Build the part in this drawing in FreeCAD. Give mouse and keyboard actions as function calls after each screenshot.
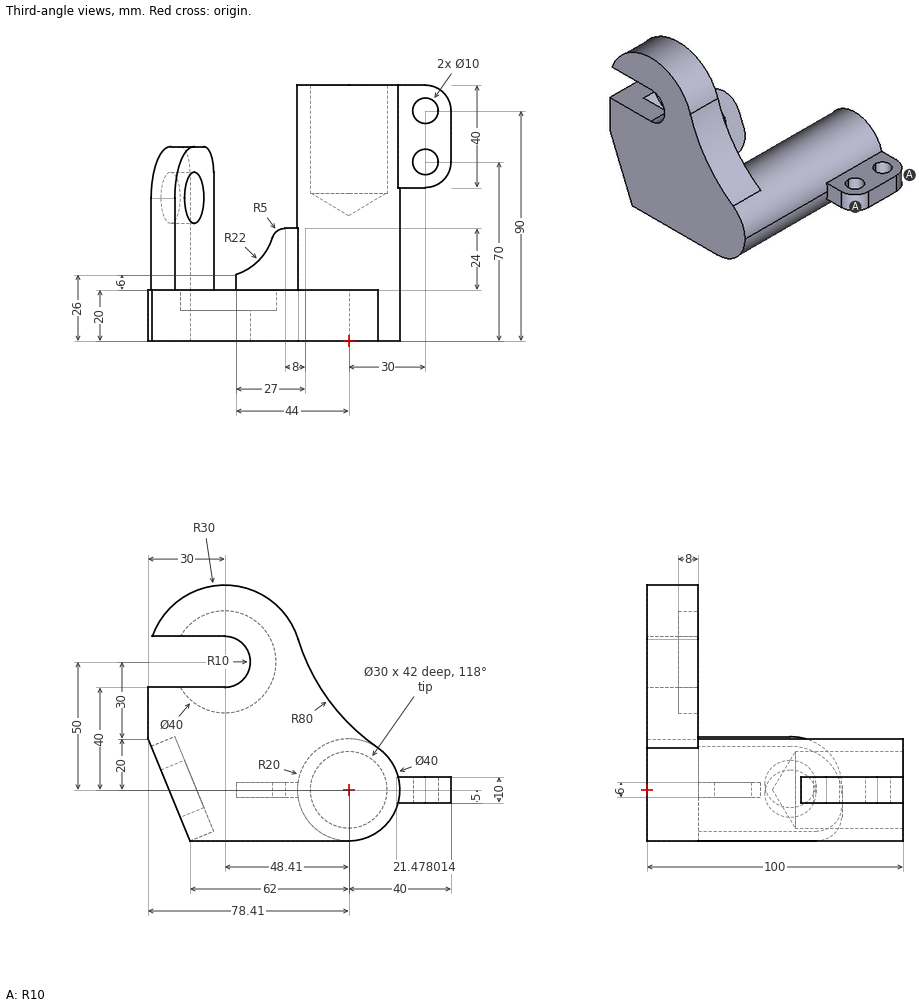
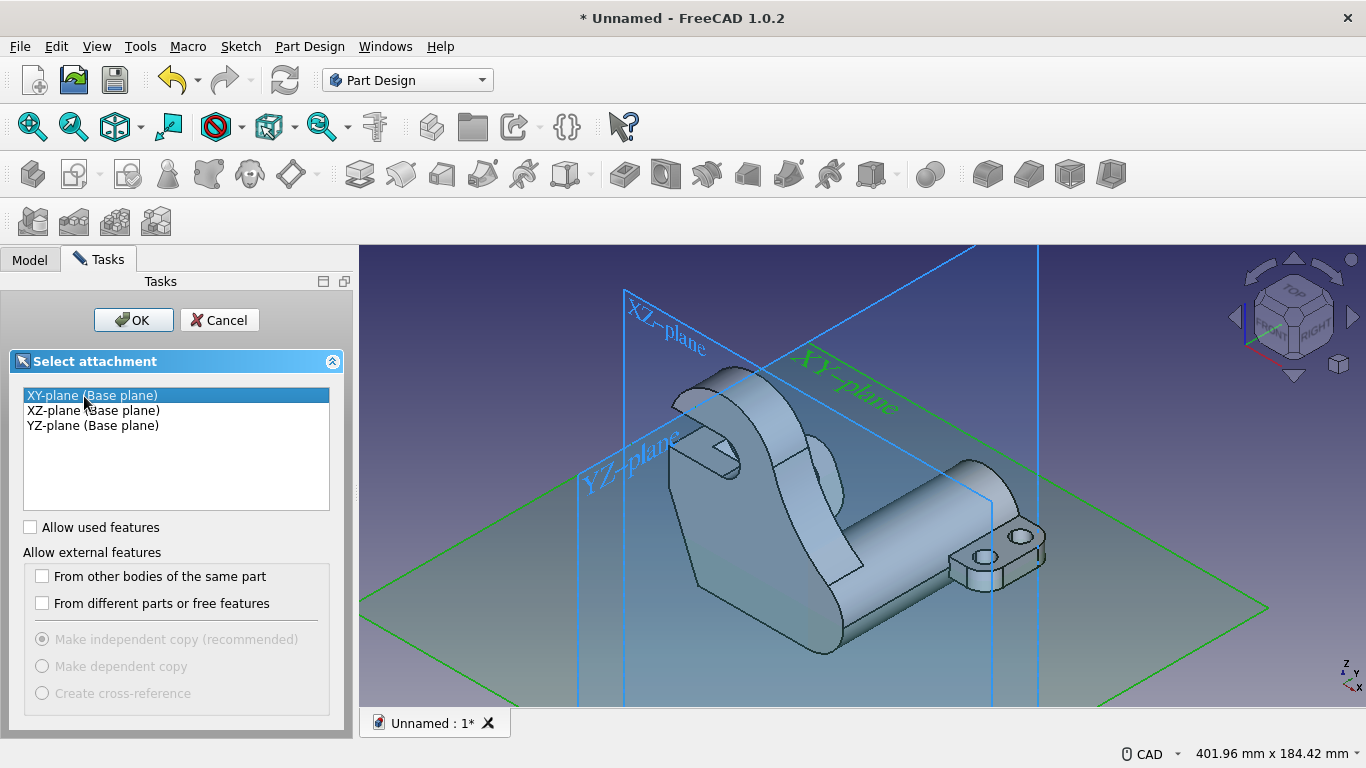
click(134, 320)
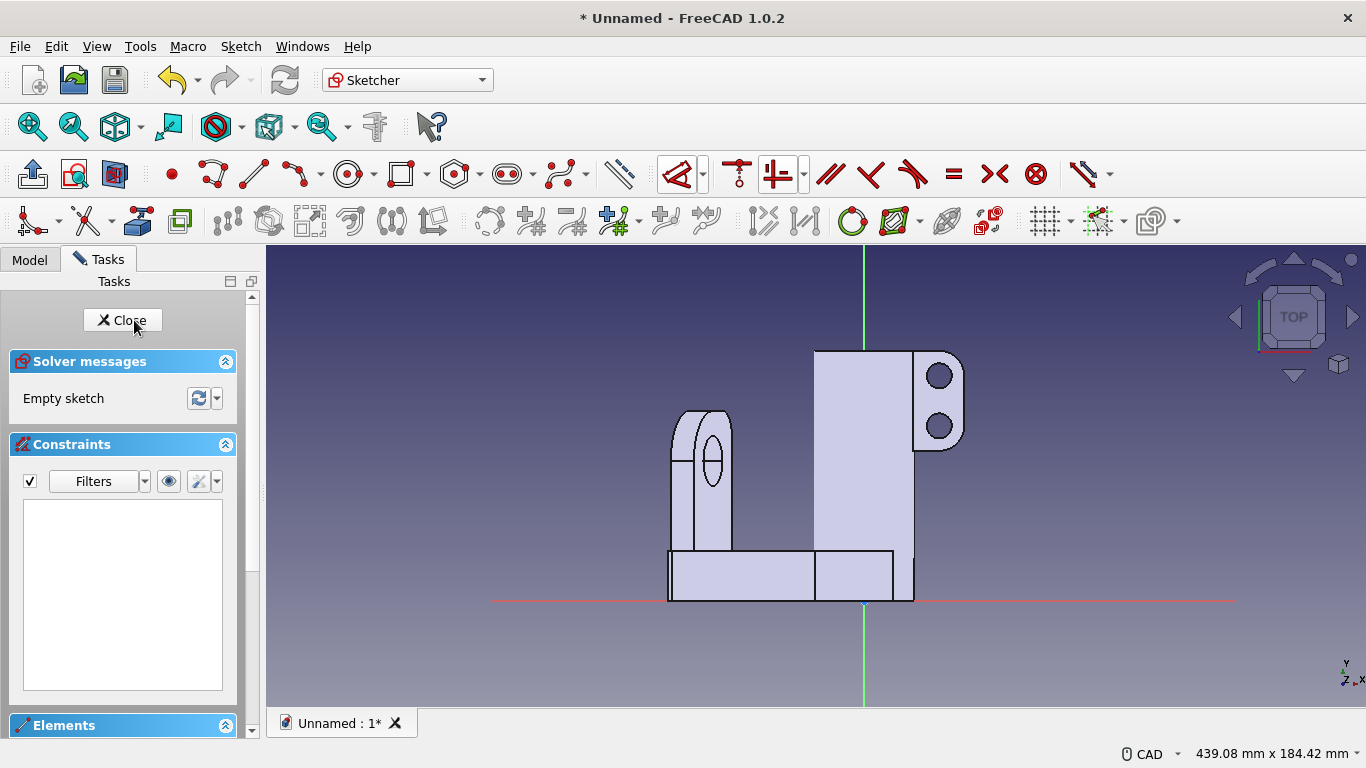
key(q)
key(s)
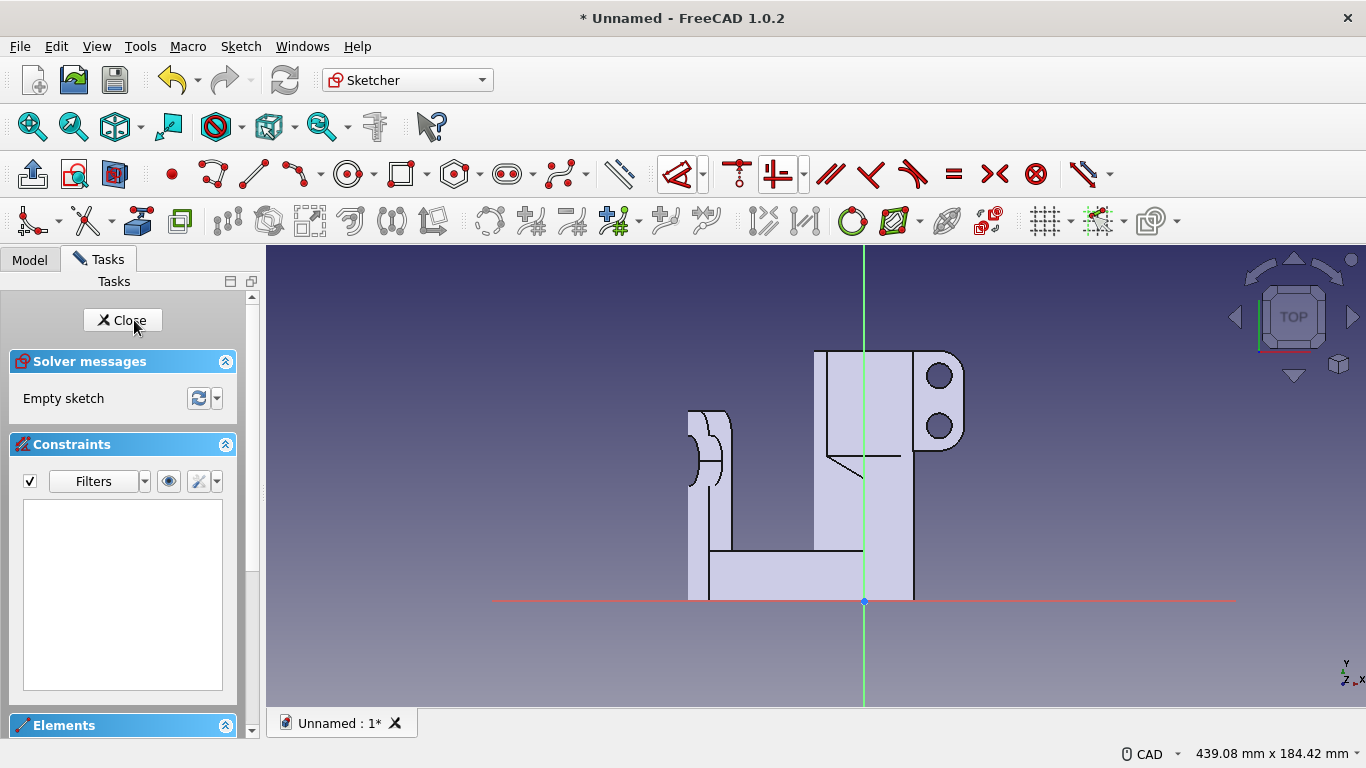
scroll(845, 587, up, 5)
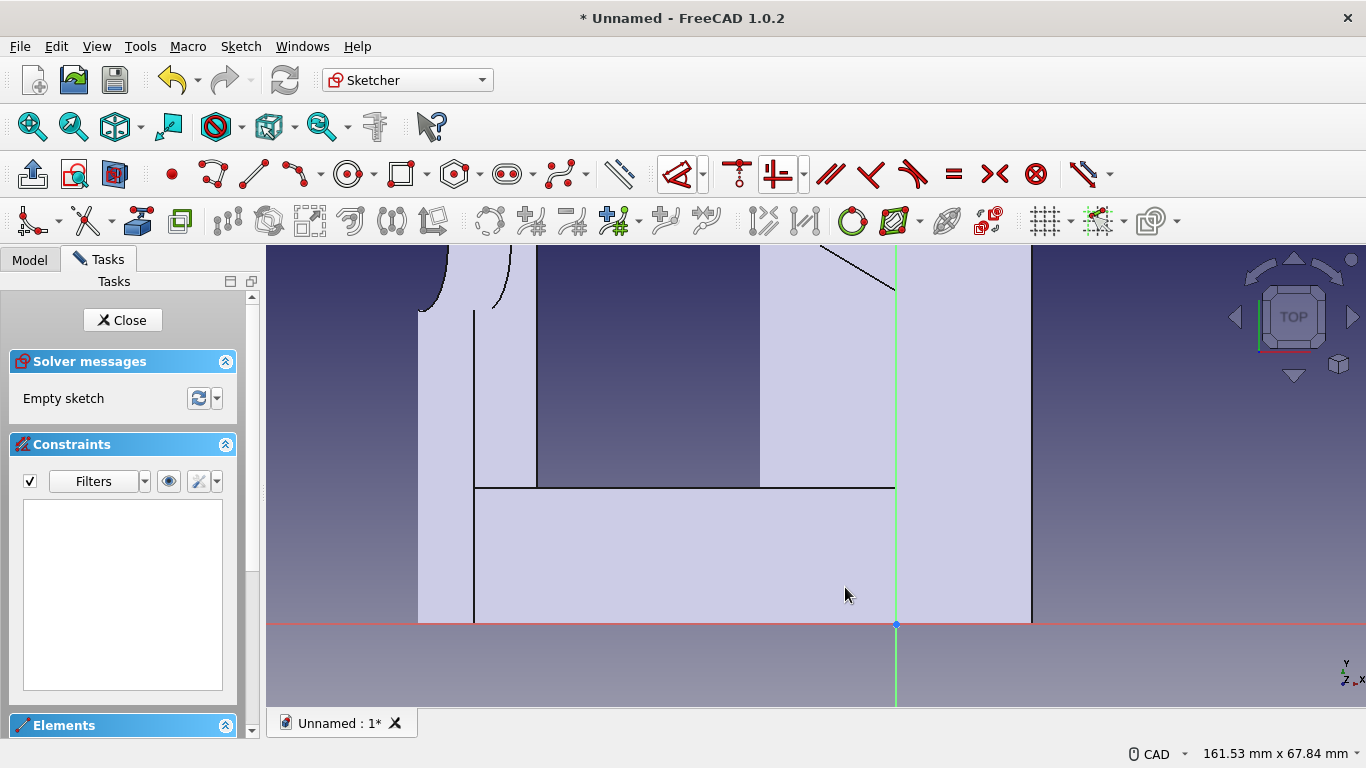
click(213, 174)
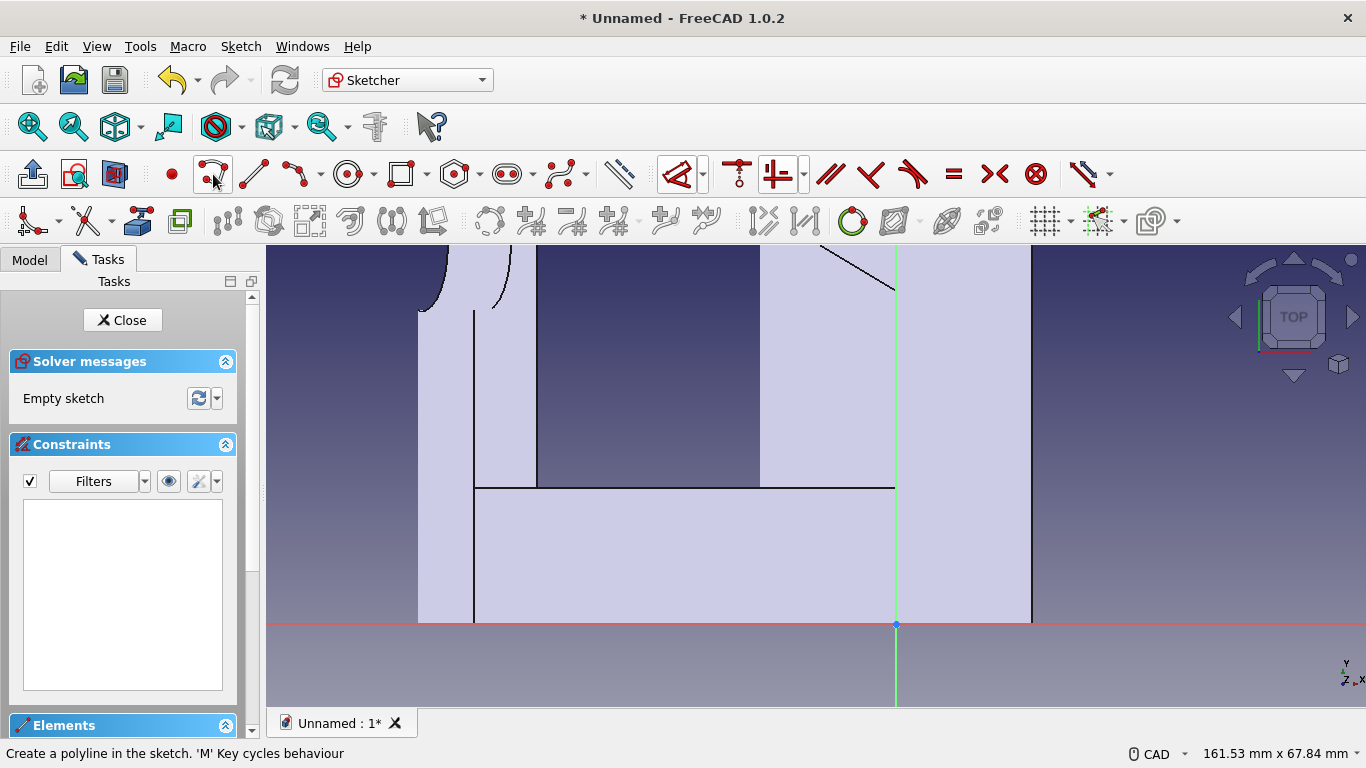
click(596, 447)
click(596, 488)
click(780, 488)
click(780, 325)
click(726, 325)
right_click(726, 325)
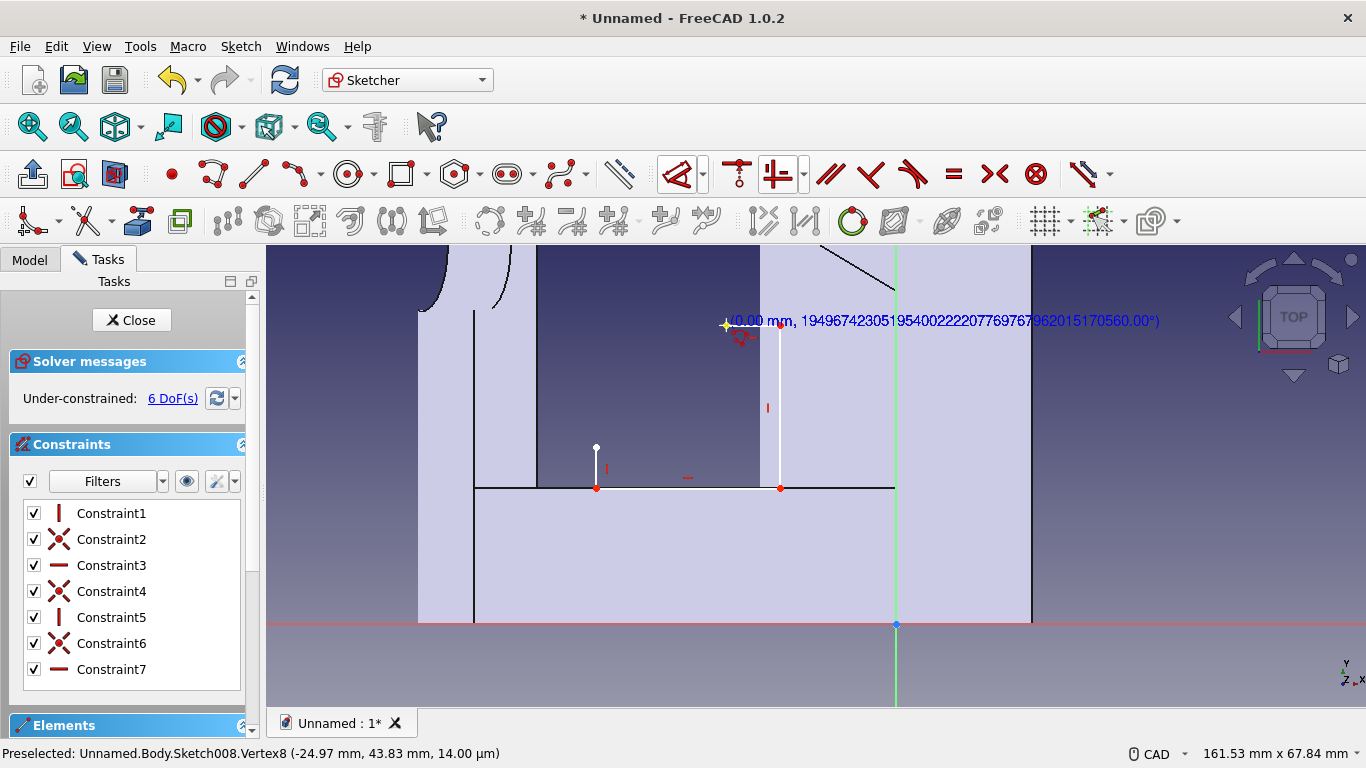
key(g)
key(3)
key(a)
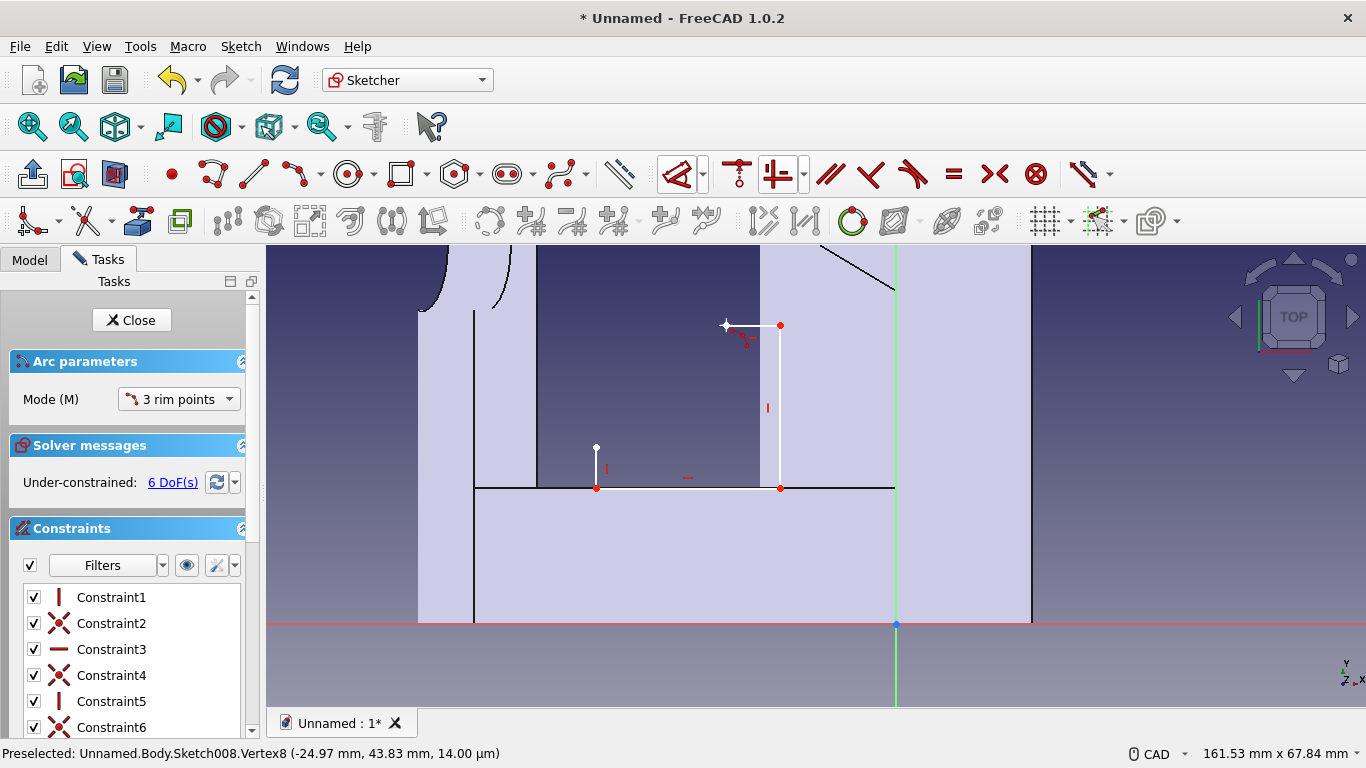
click(726, 326)
click(693, 349)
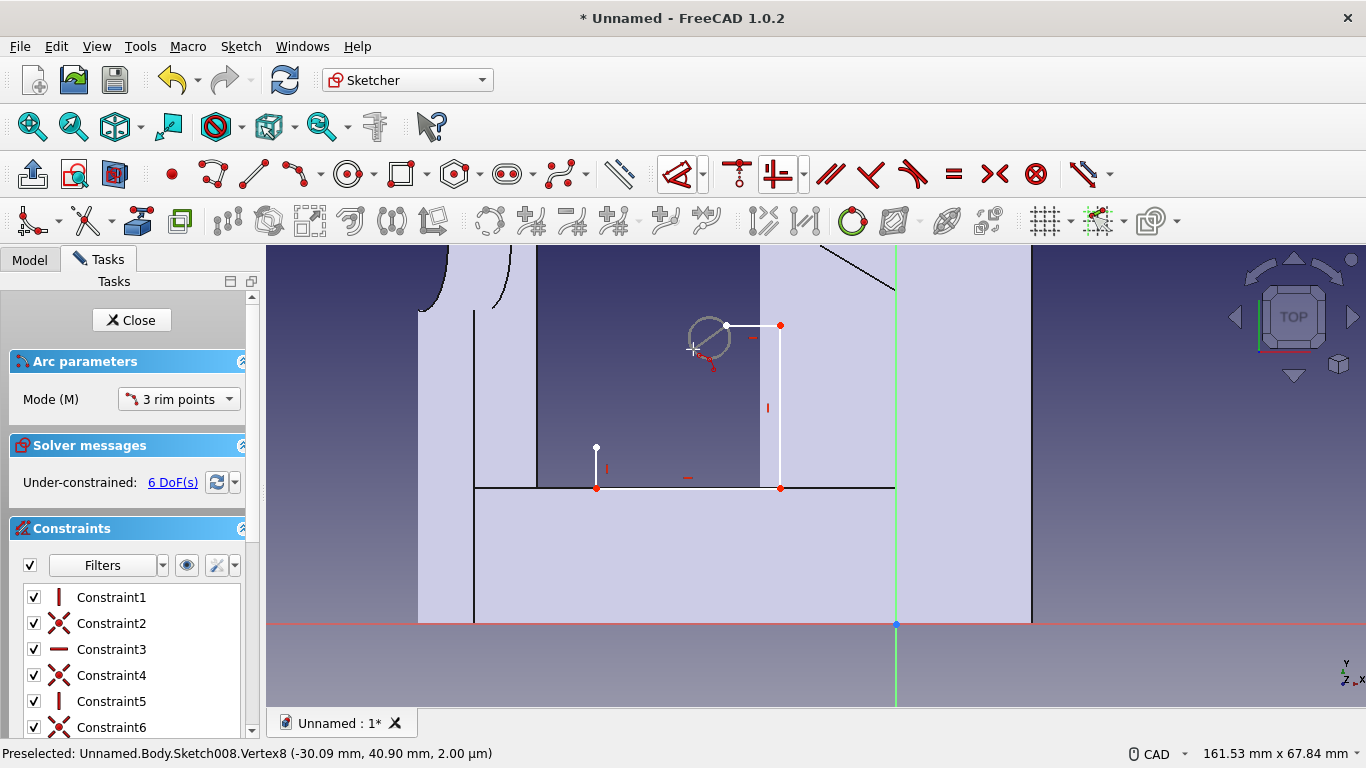
scroll(706, 332, up, 5)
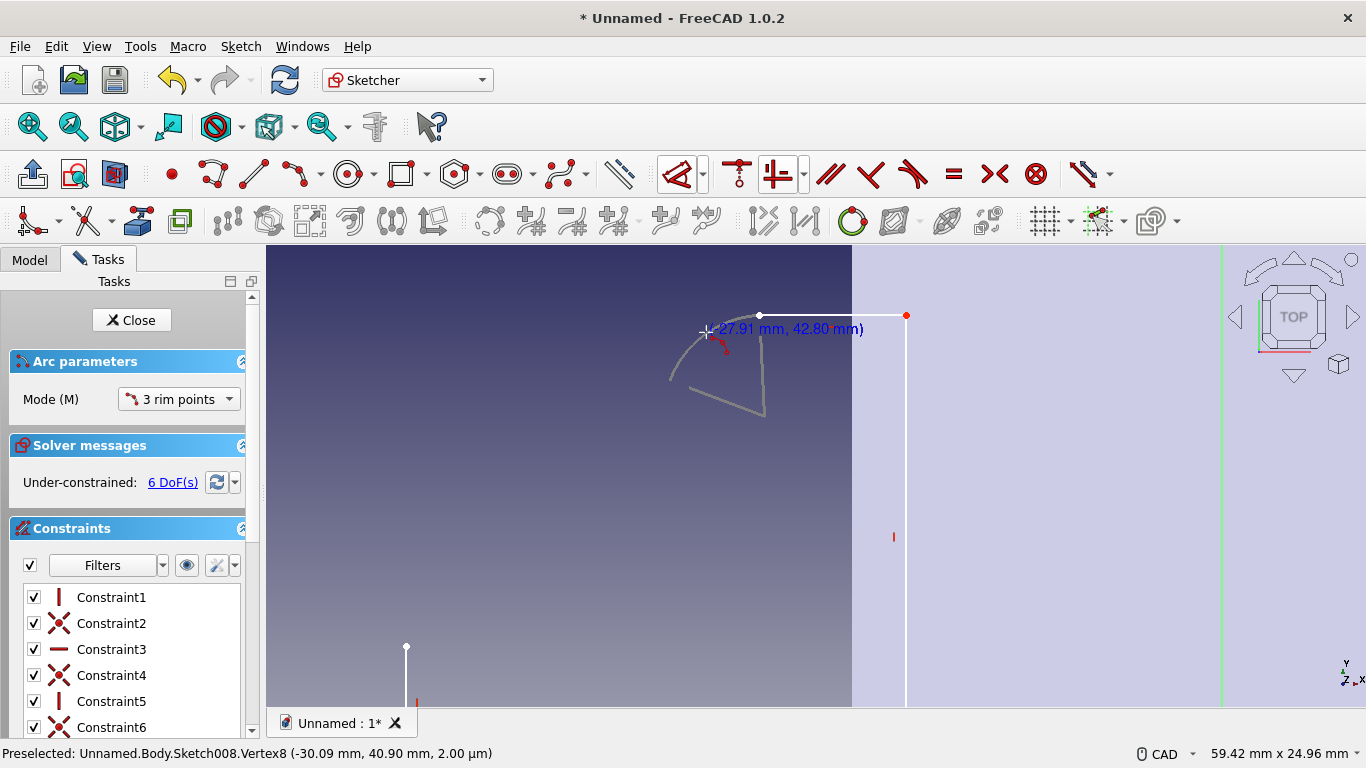
click(704, 330)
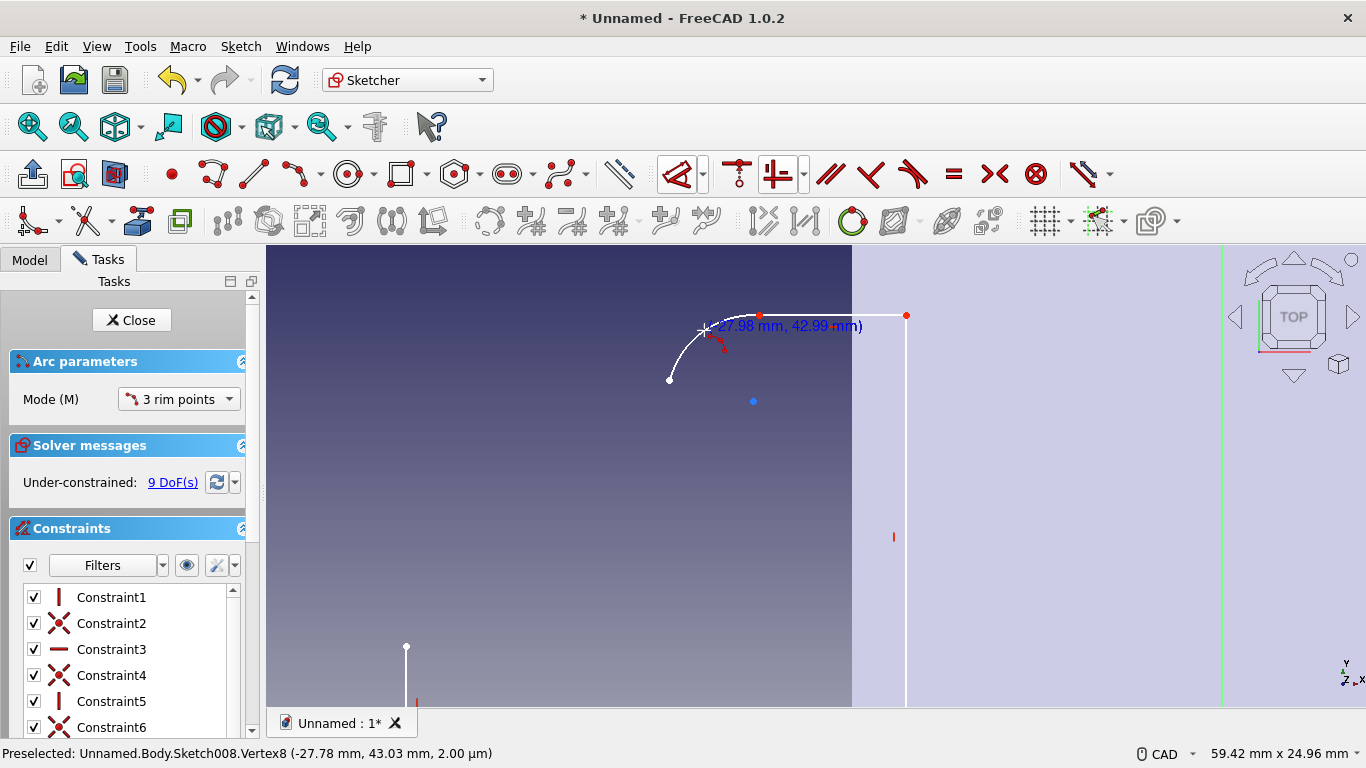
click(670, 381)
click(406, 647)
click(572, 544)
key(Escape)